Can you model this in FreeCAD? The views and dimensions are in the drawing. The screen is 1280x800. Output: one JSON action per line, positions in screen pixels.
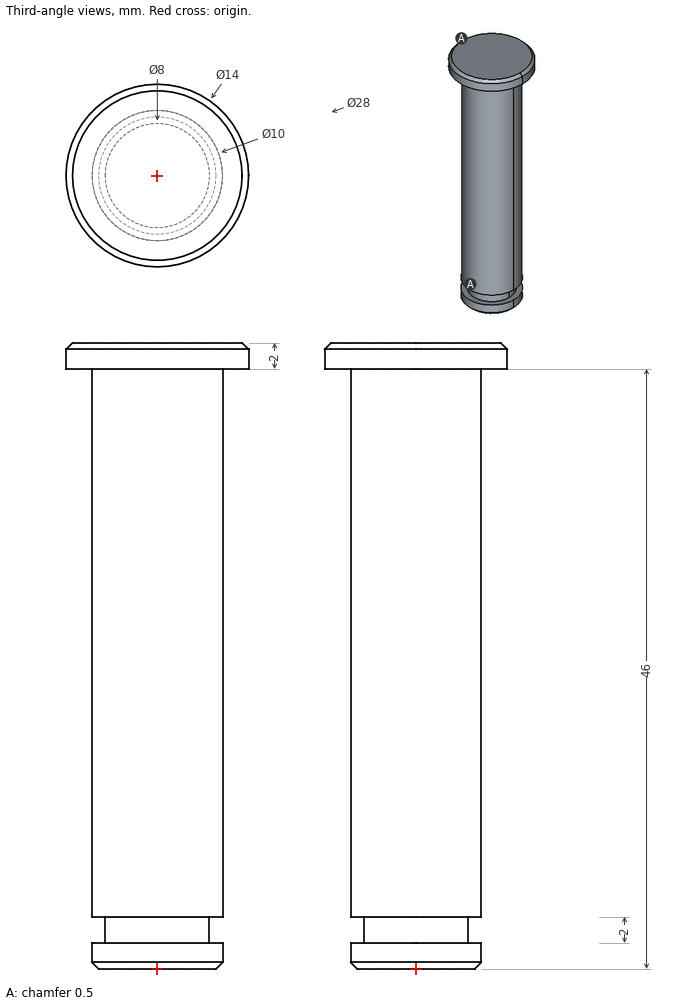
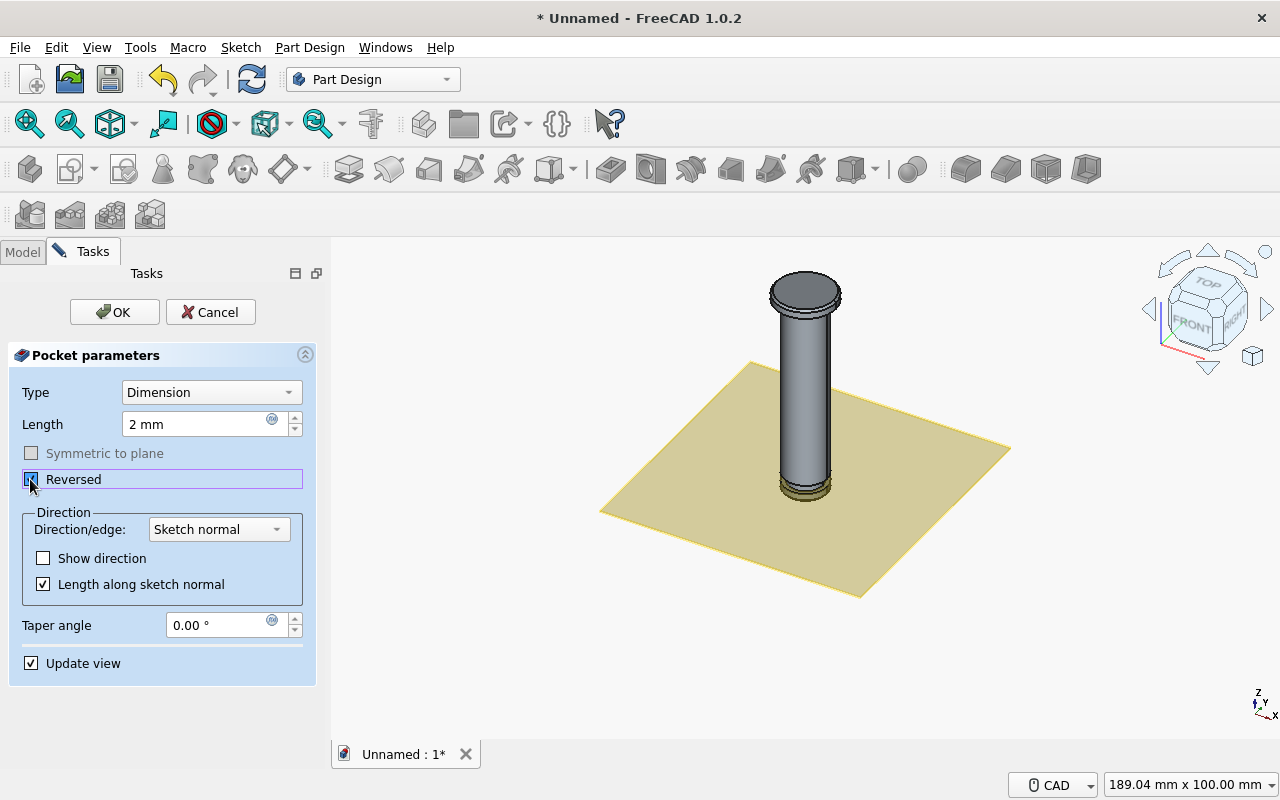
{"action": "left_click", "coordinate": [115, 312]}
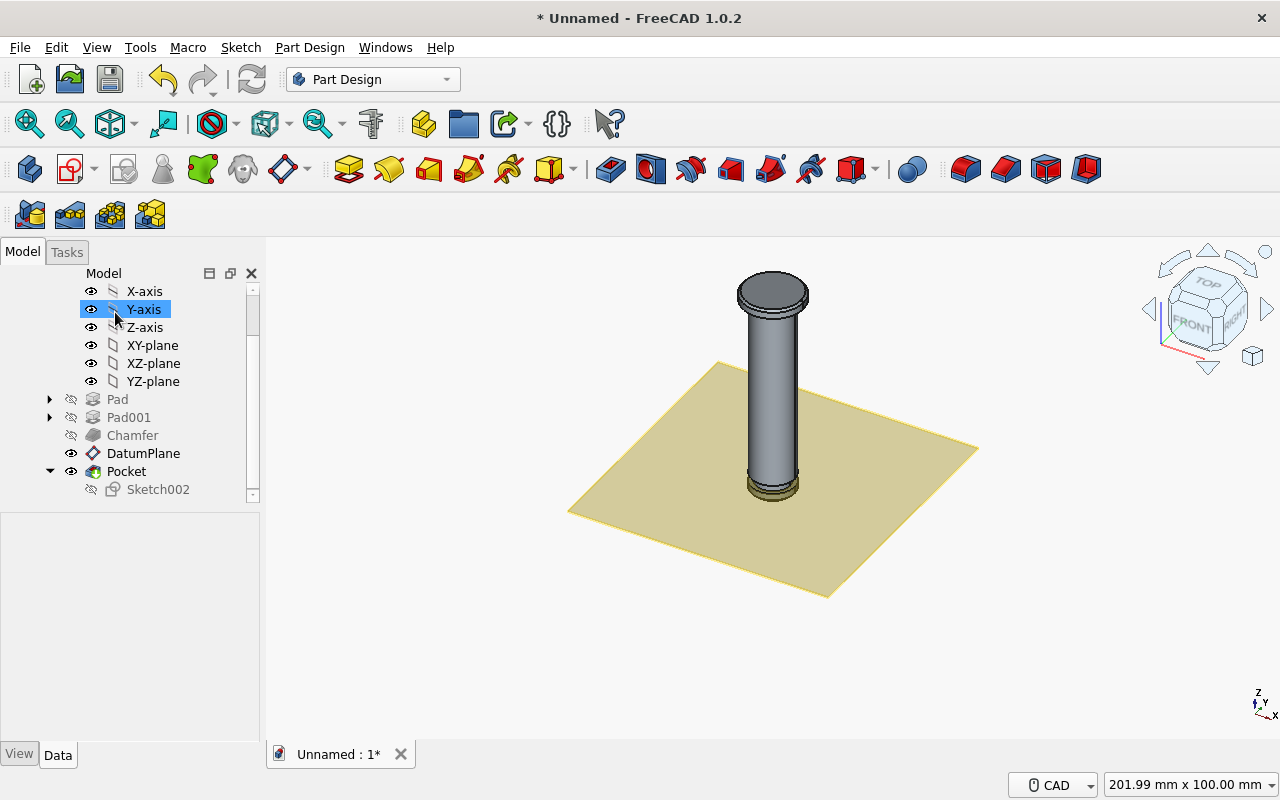
{"action": "left_click", "coordinate": [116, 453]}
{"action": "key", "text": "space"}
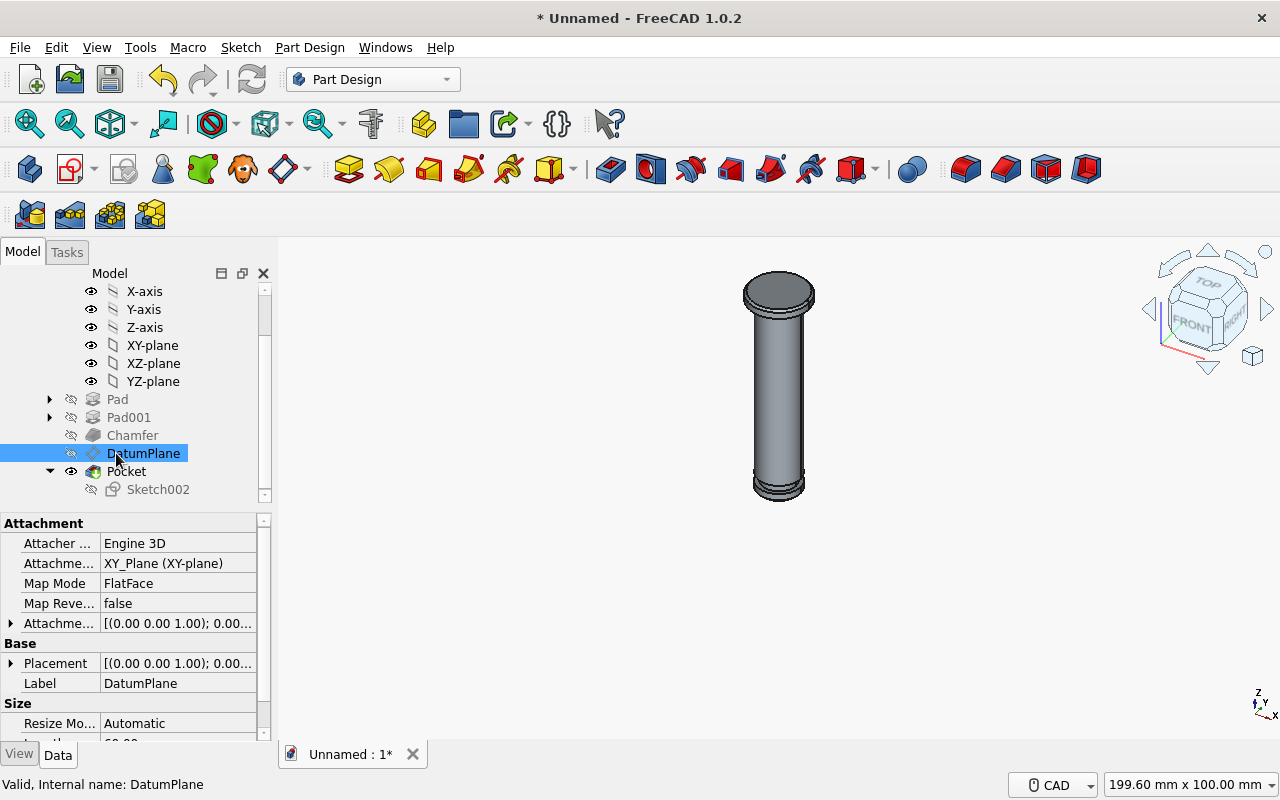
{"action": "key", "text": "0"}